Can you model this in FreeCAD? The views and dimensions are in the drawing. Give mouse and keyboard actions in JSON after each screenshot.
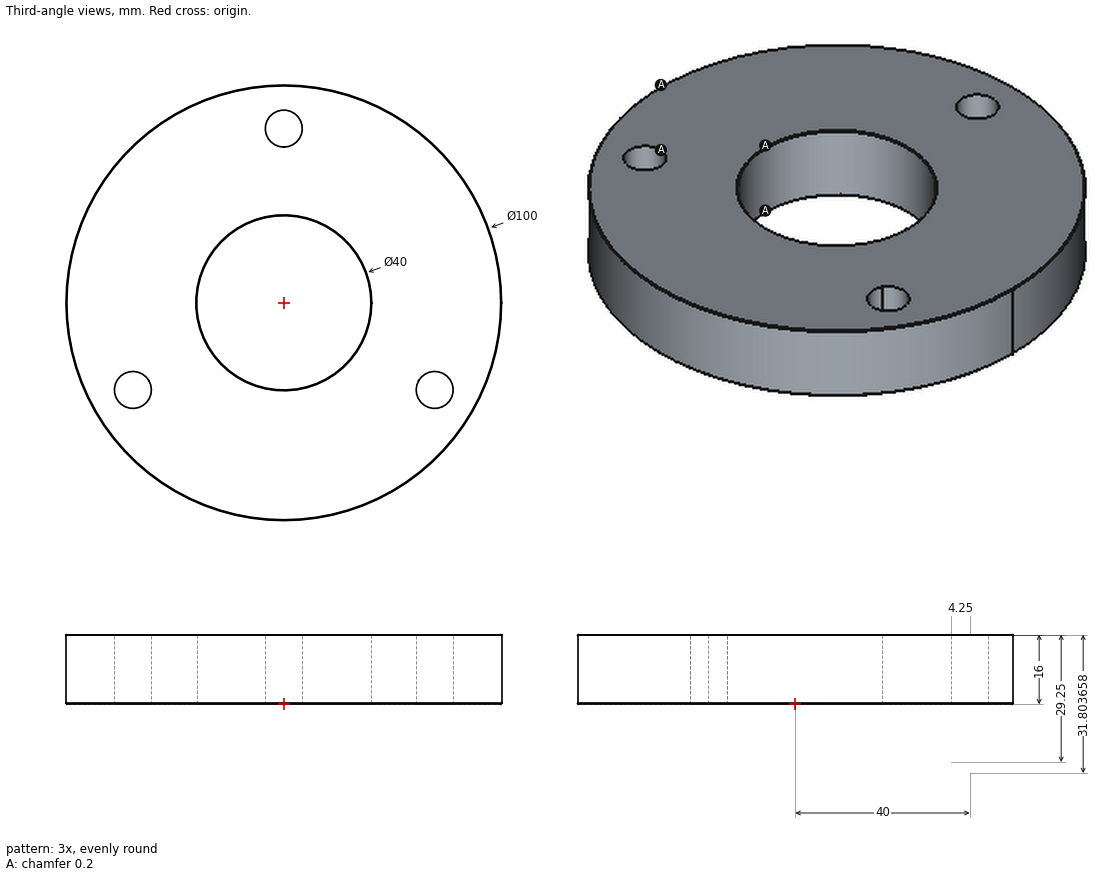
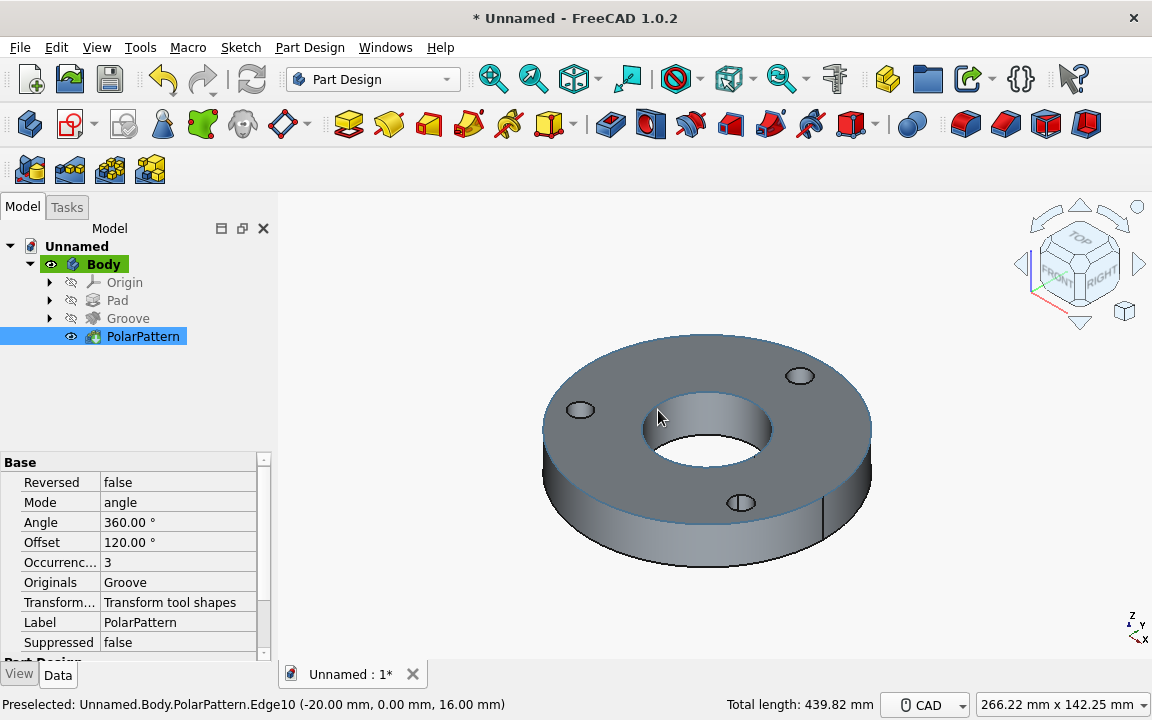
{"action": "key", "text": "2"}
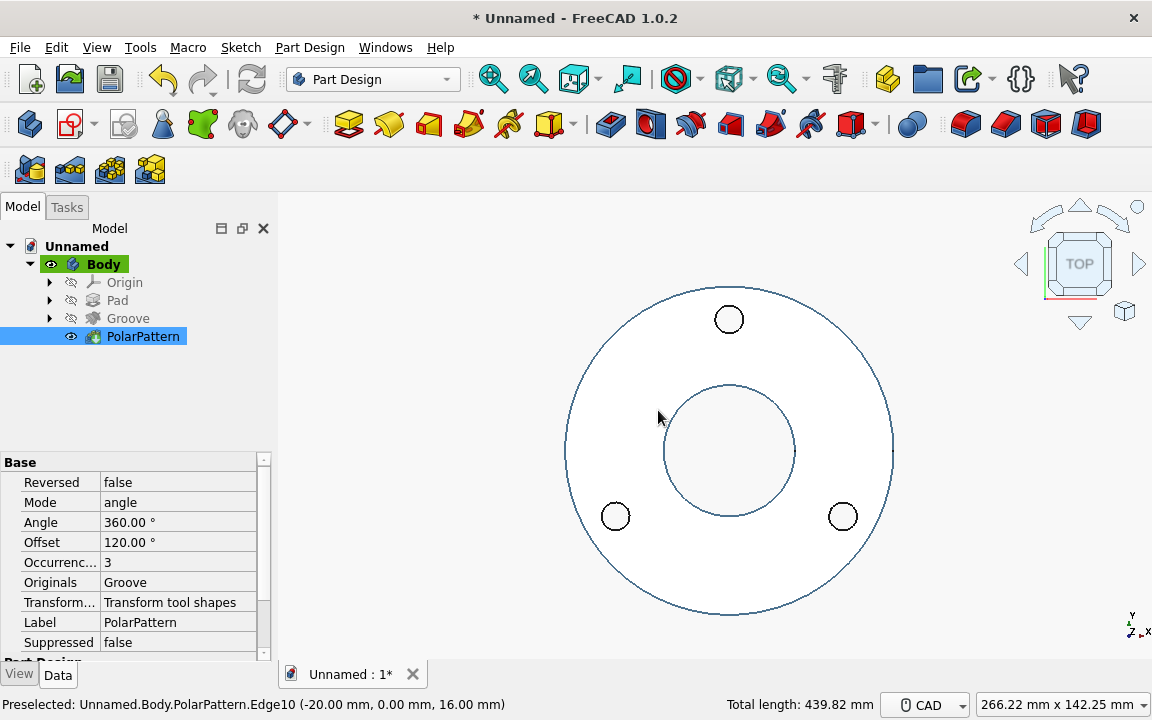
{"action": "key", "text": "1"}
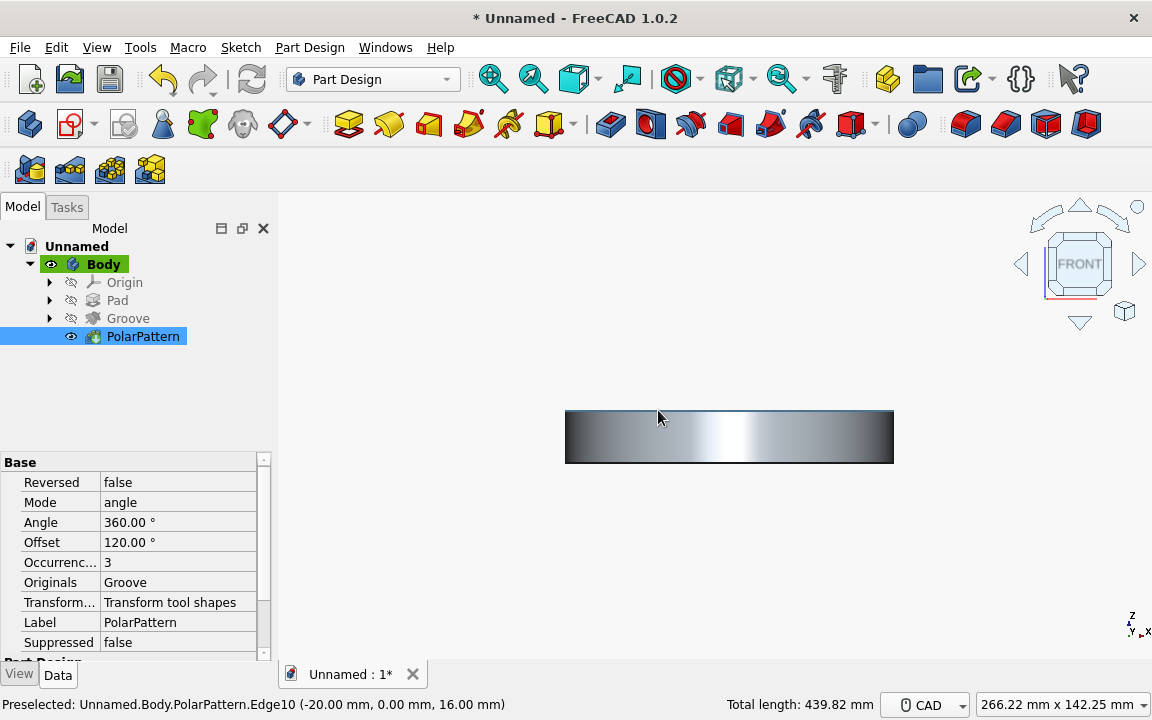
{"action": "left_click", "coordinate": [494, 80]}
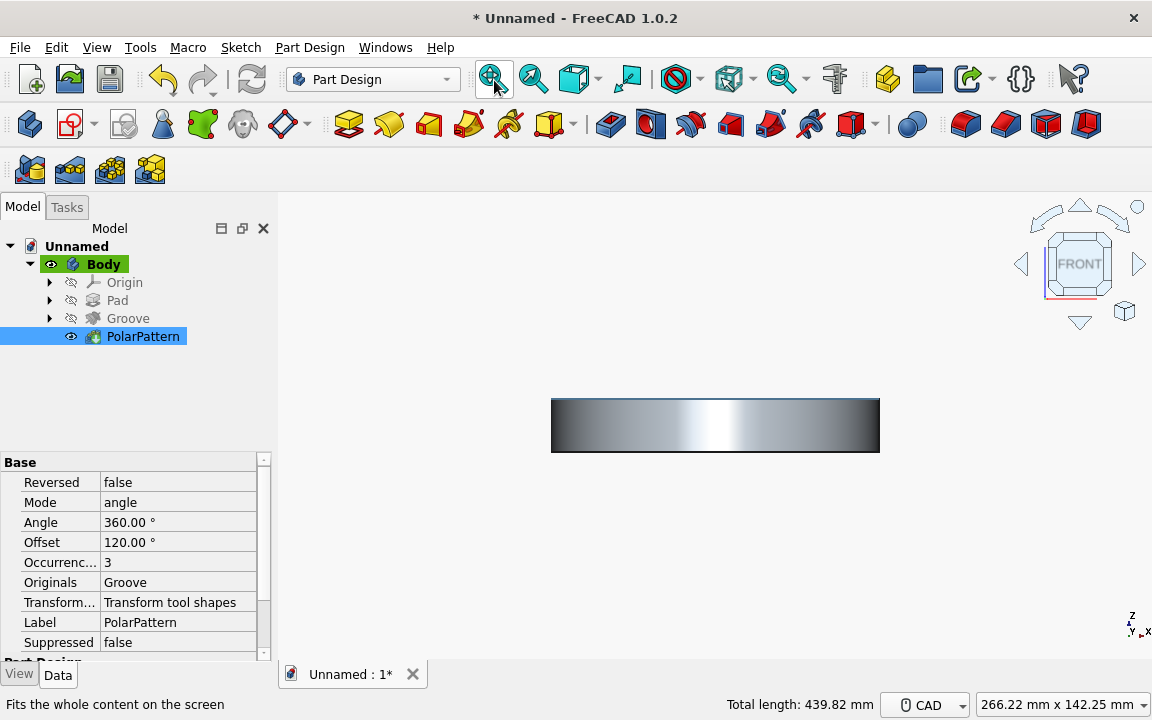
{"action": "left_click", "coordinate": [582, 451], "text": "ctrl"}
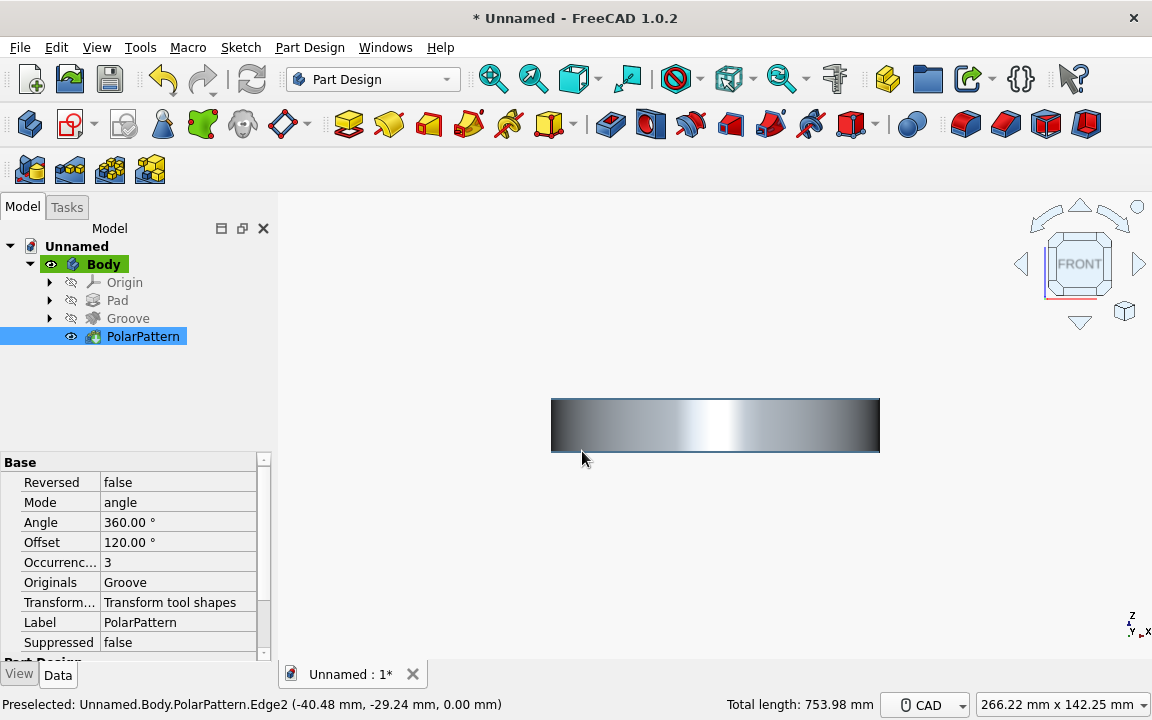
{"action": "key", "text": "3"}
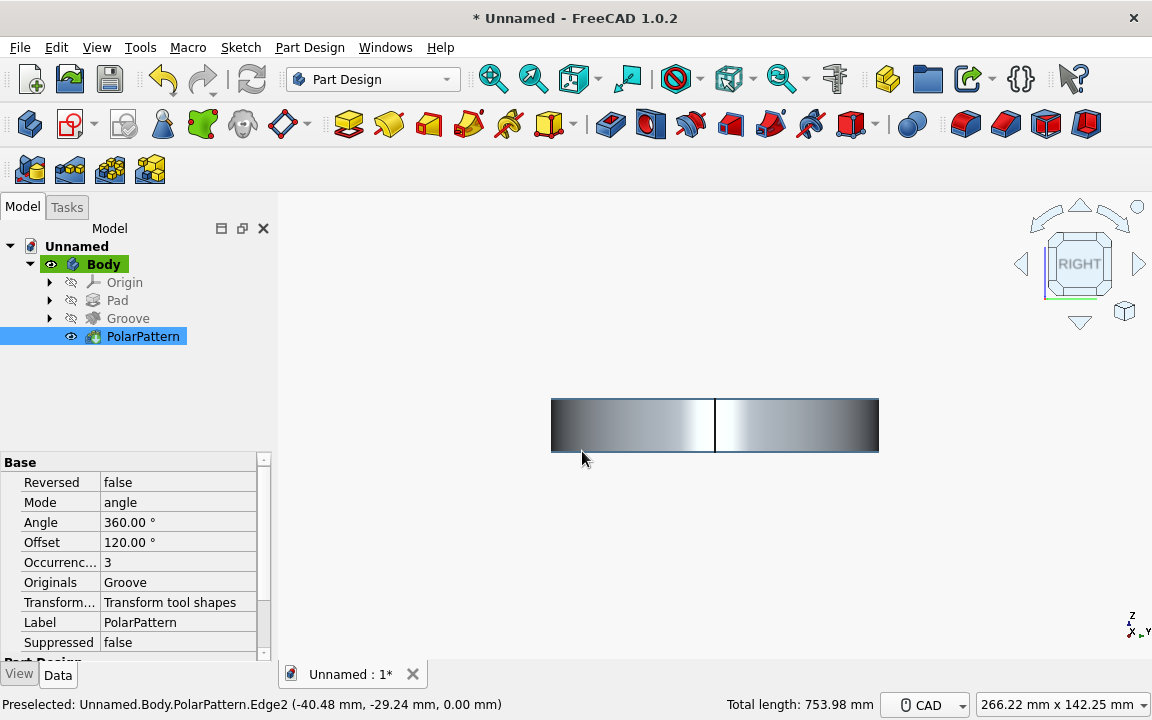
{"action": "left_click", "coordinate": [494, 80]}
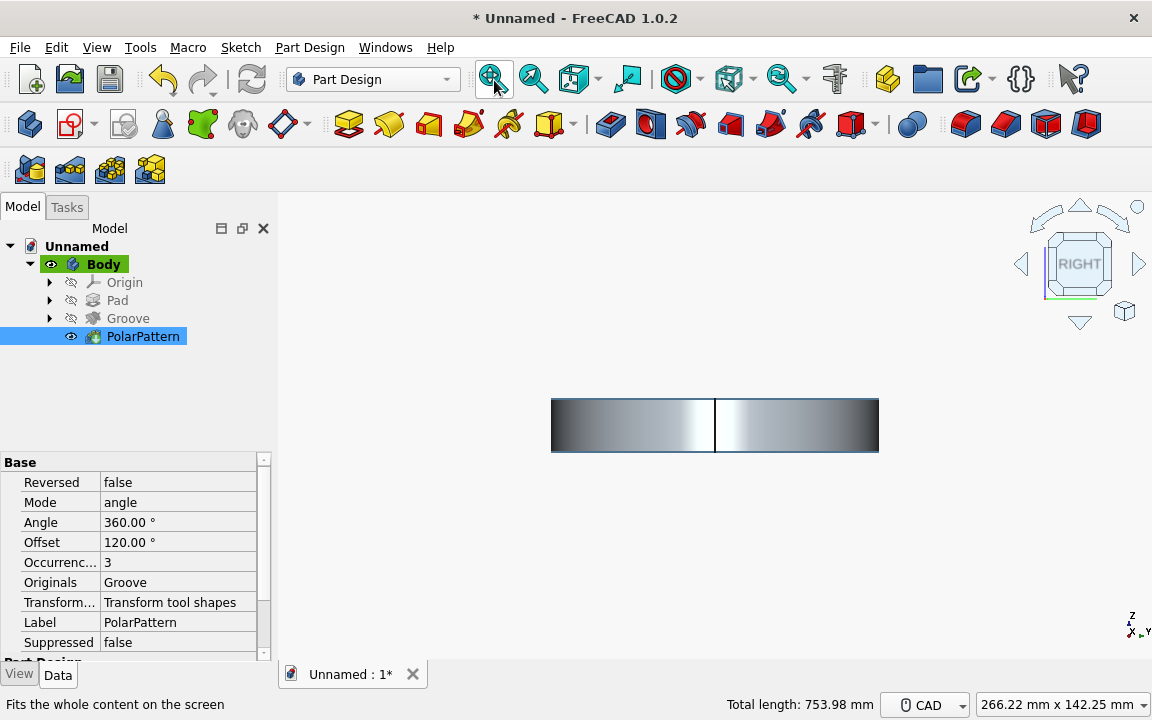
{"action": "key", "text": "5"}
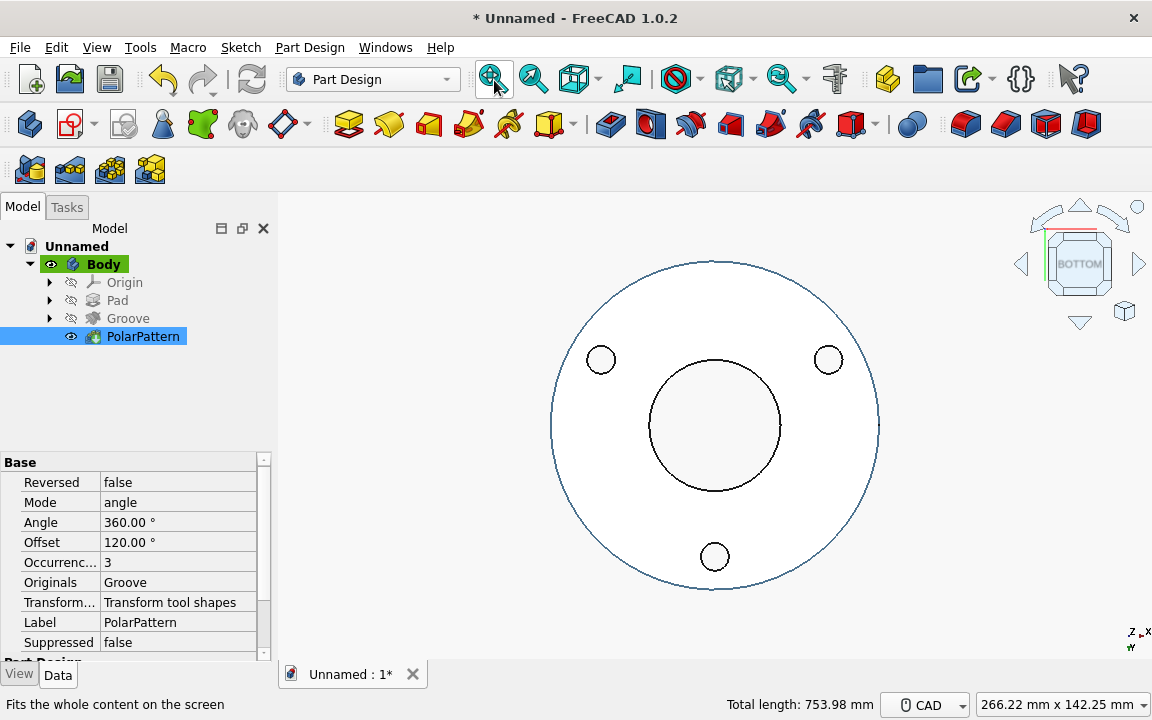
{"action": "left_click", "coordinate": [662, 386], "text": "ctrl"}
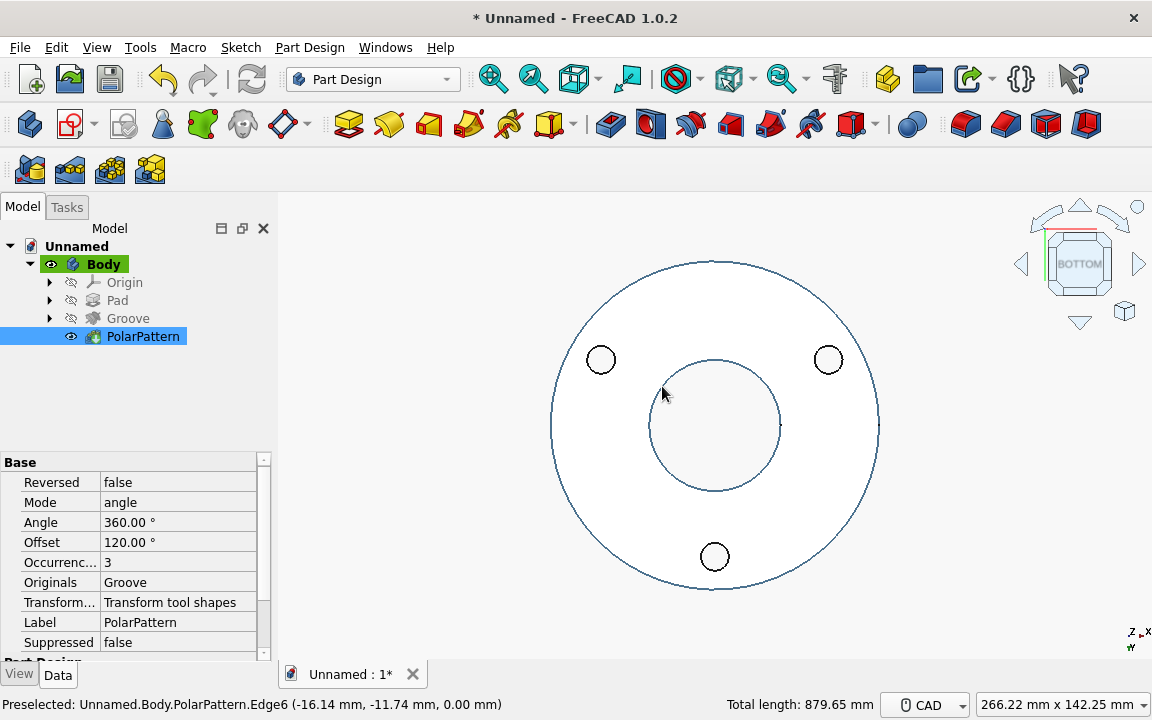
{"action": "left_click", "coordinate": [1006, 124]}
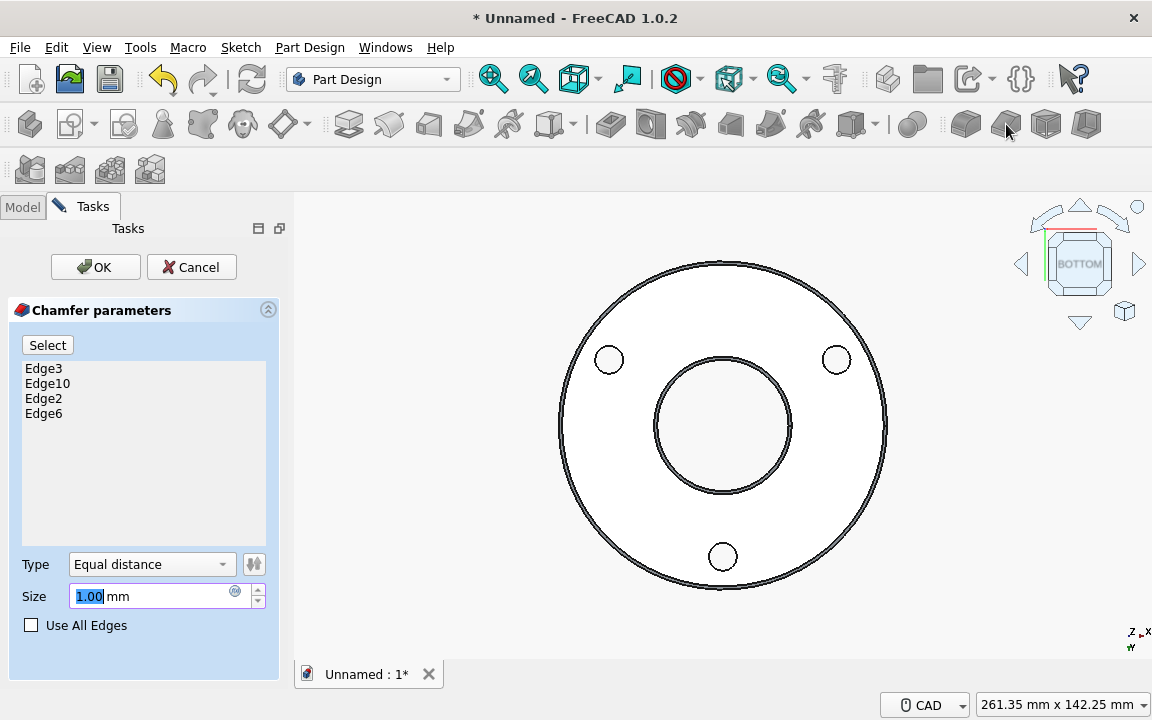
{"action": "type", "text": "0.2"}
{"action": "key", "text": "Tab"}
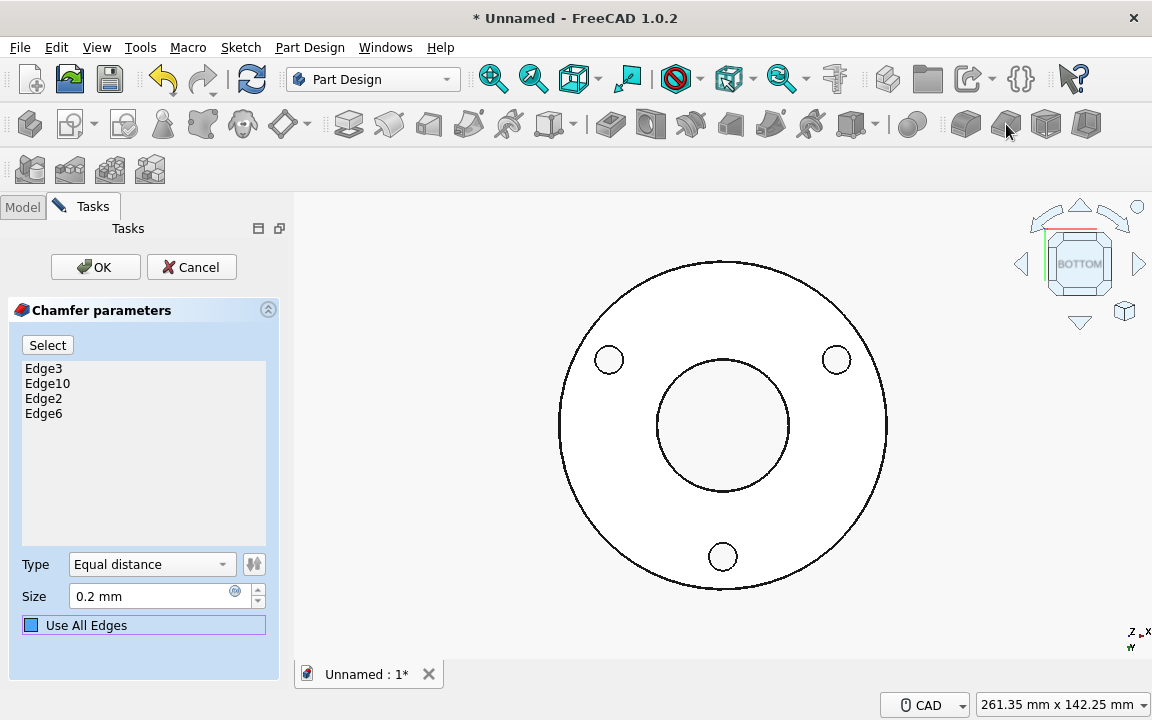
{"action": "left_click", "coordinate": [96, 267]}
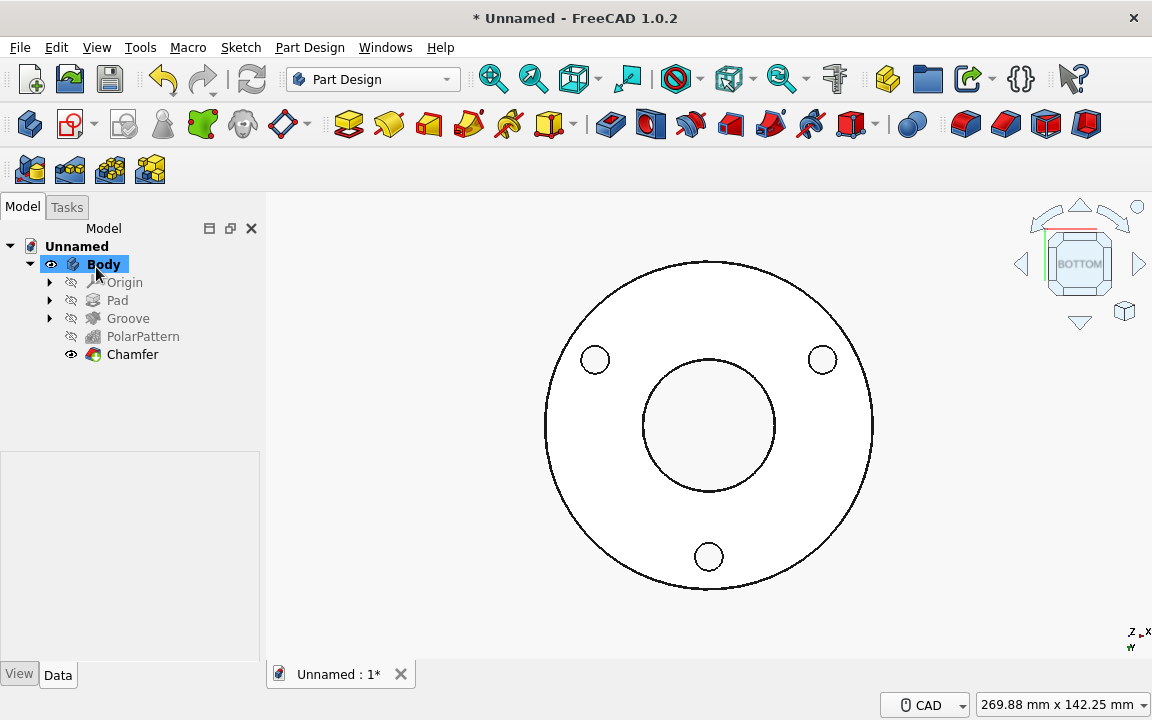
{"action": "key", "text": "0"}